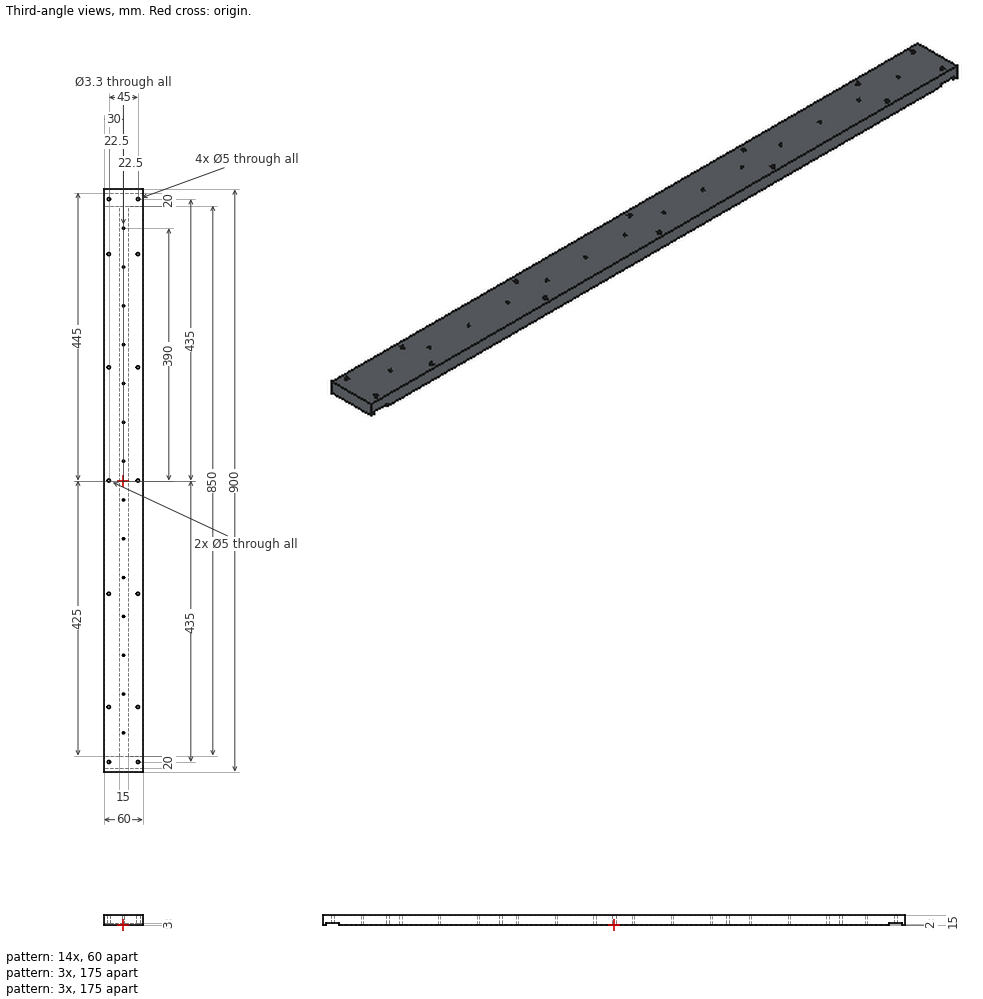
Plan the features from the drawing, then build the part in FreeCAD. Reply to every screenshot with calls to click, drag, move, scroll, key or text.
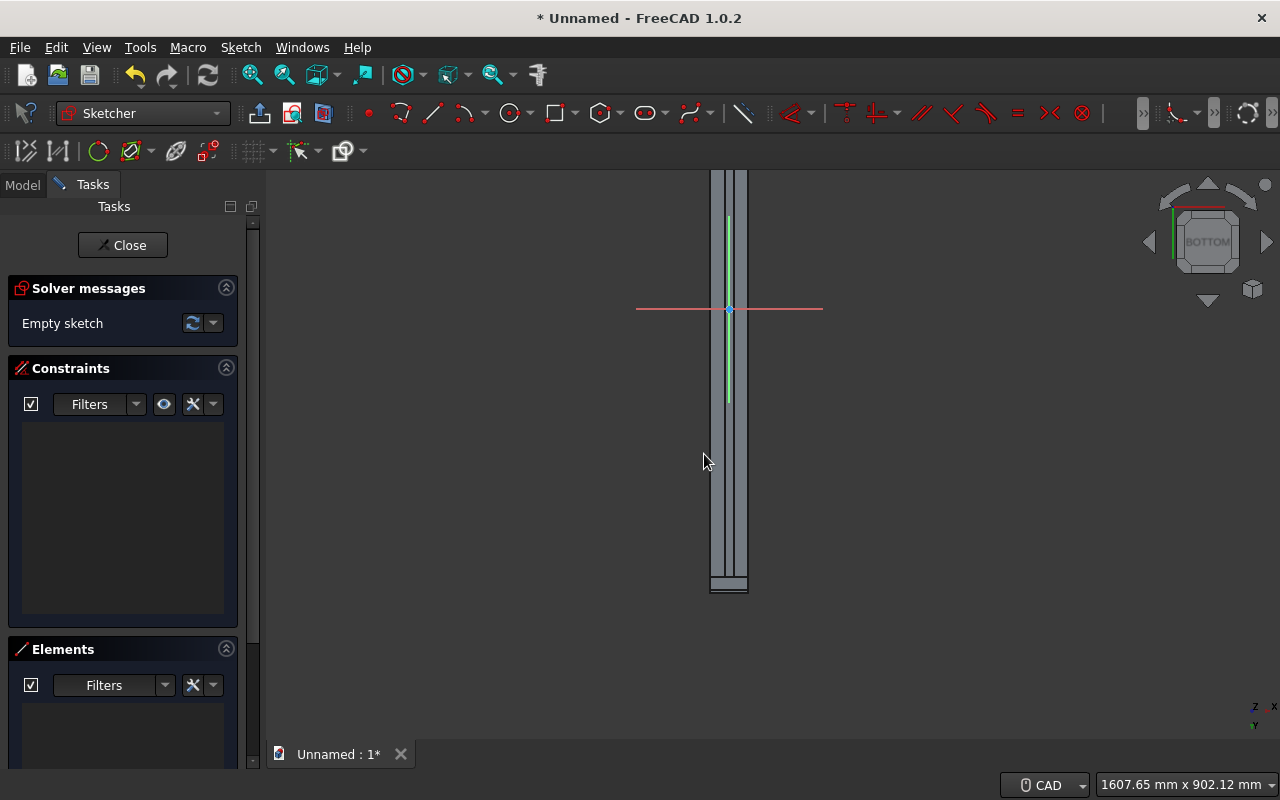
scroll(731, 560, up, 15)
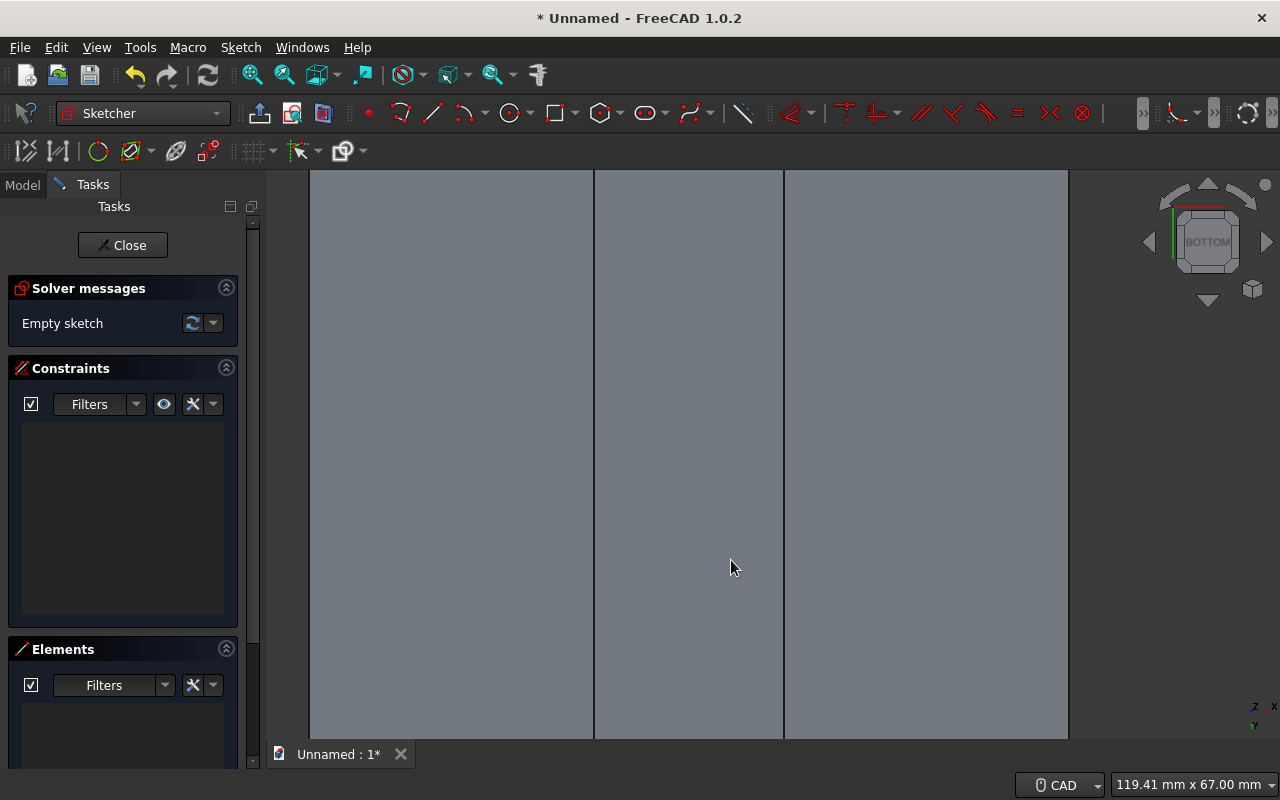
scroll(687, 446, up, 11)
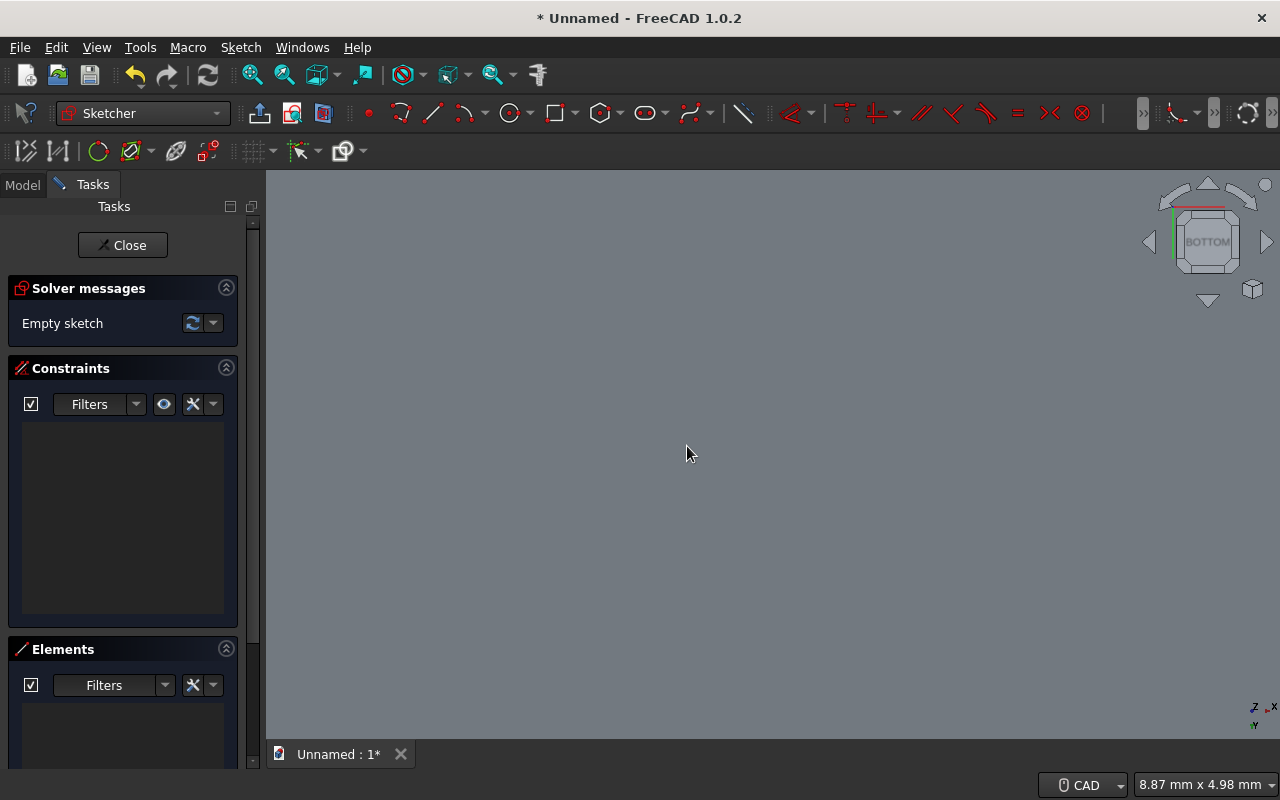
key(g)
key(c)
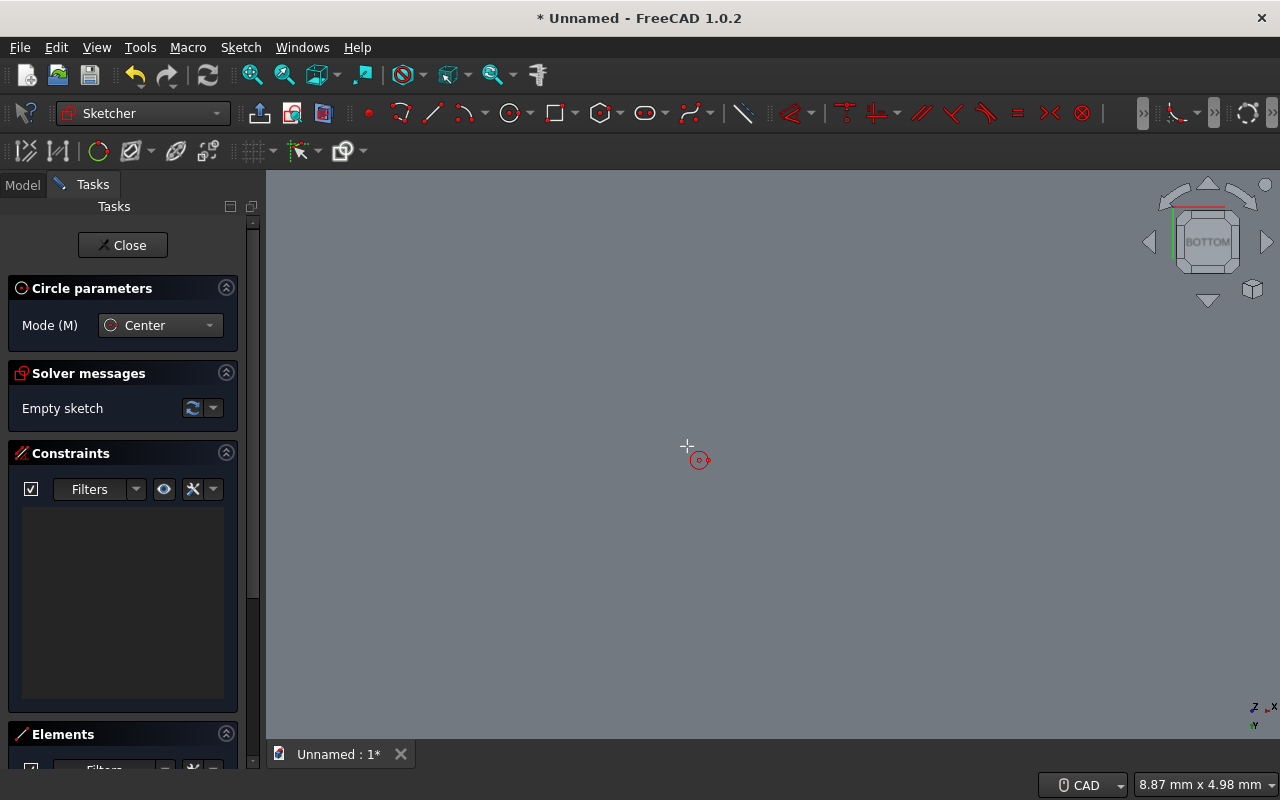
click(705, 449)
move(838, 316)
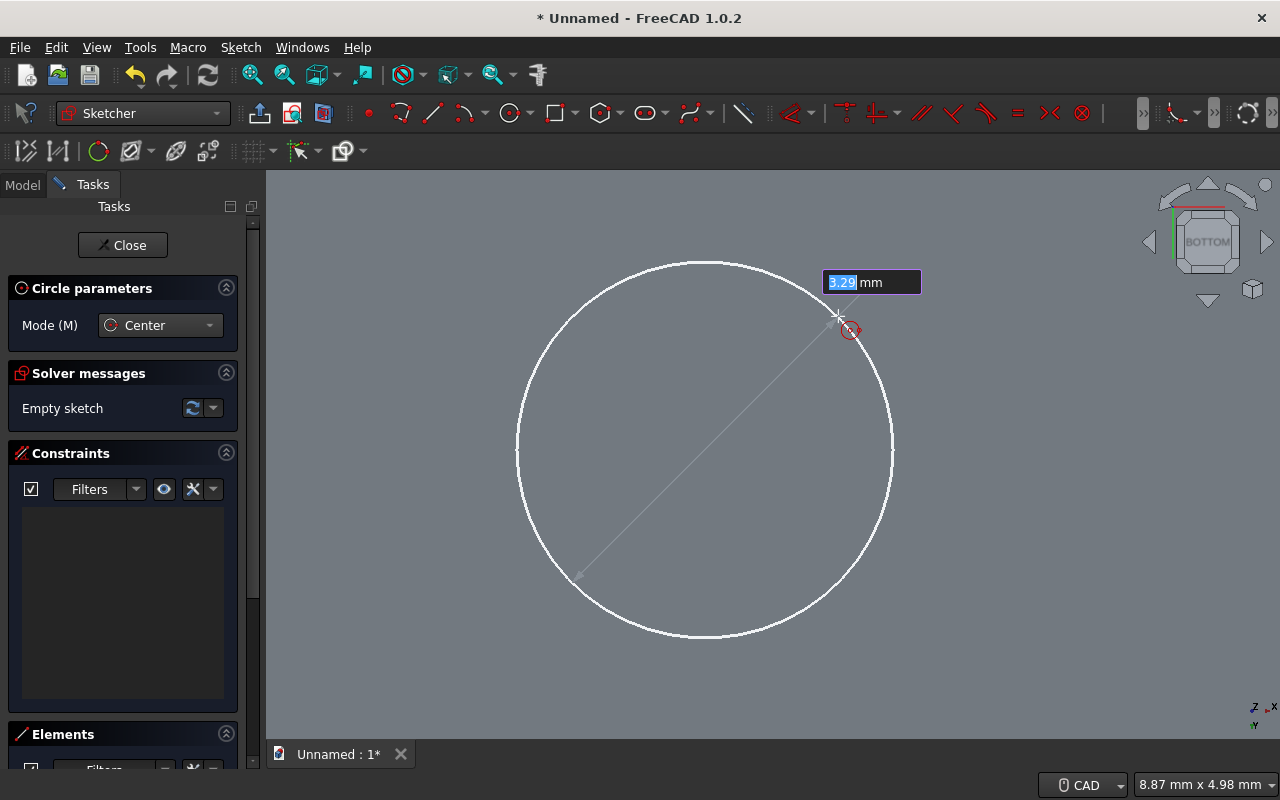
text(3.3)
key(Return)
key(Escape)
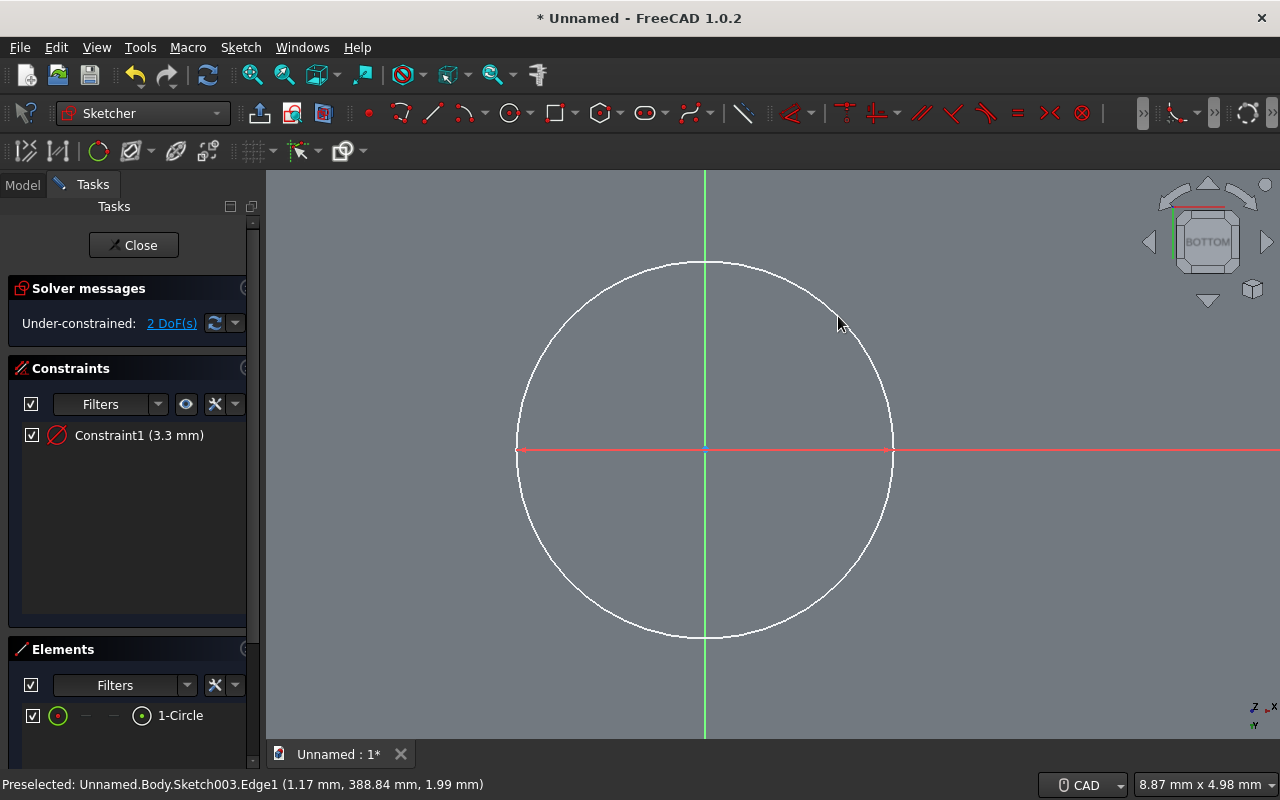
click(705, 450)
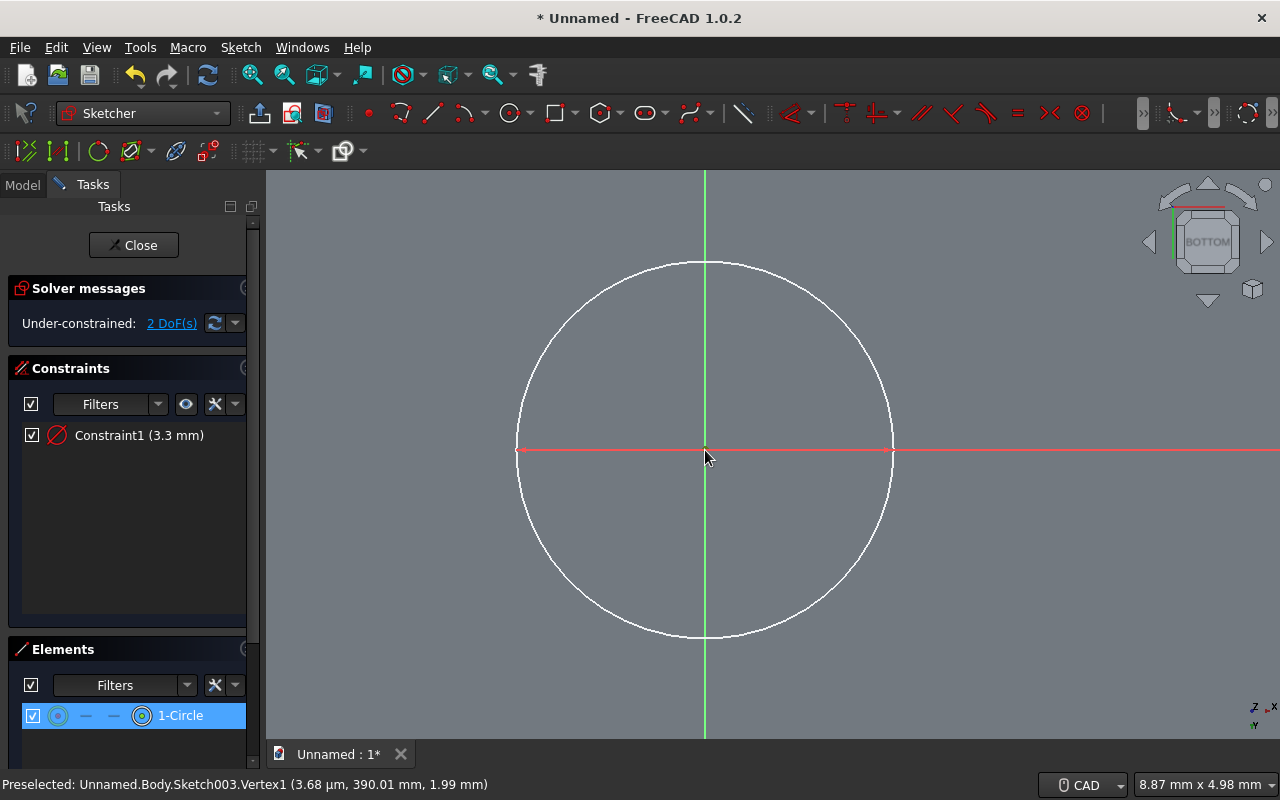
click(705, 674)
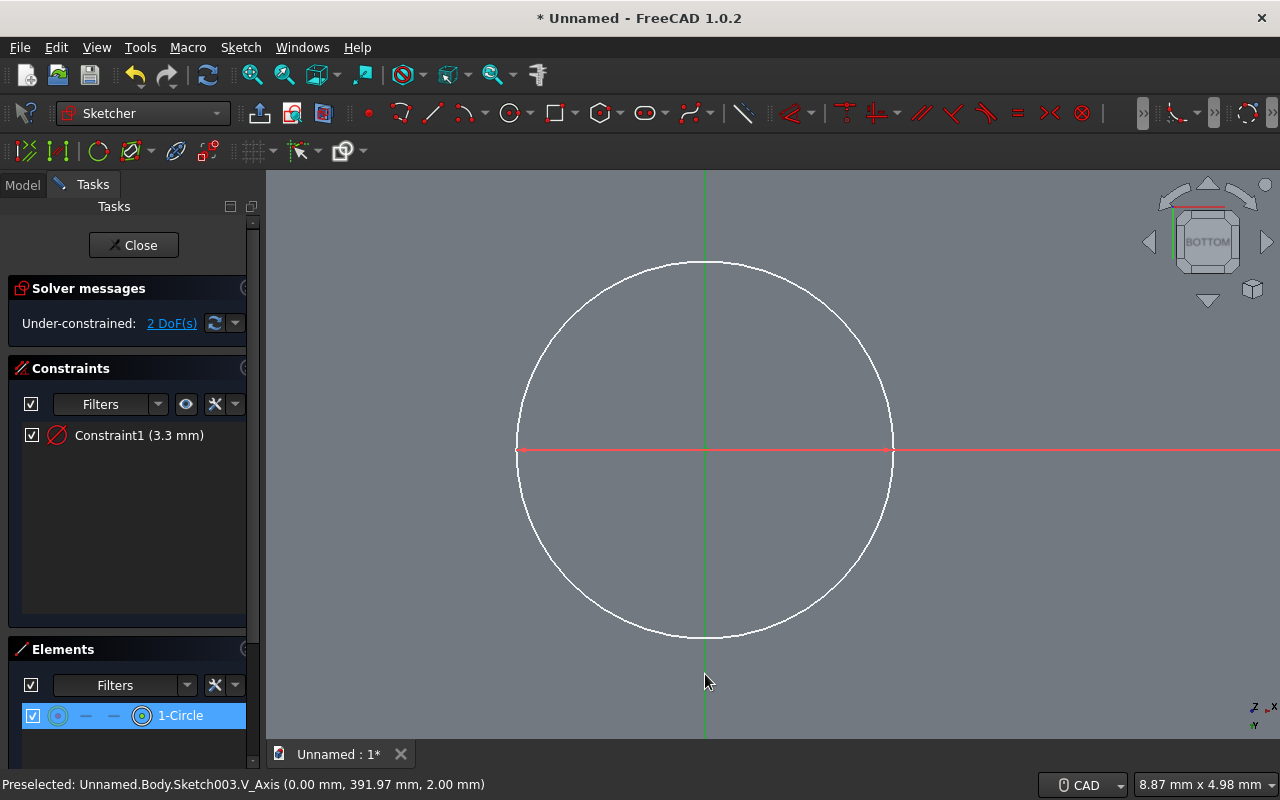
click(846, 114)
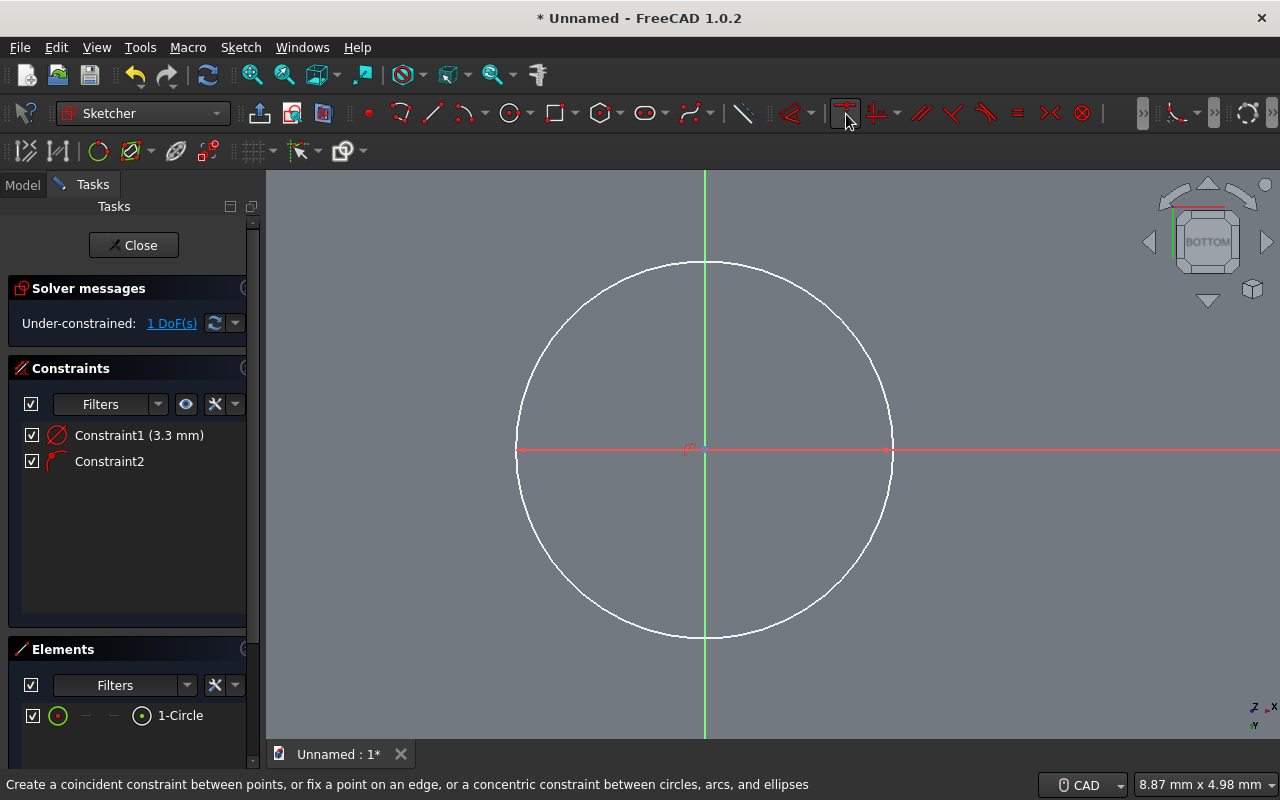
key(d)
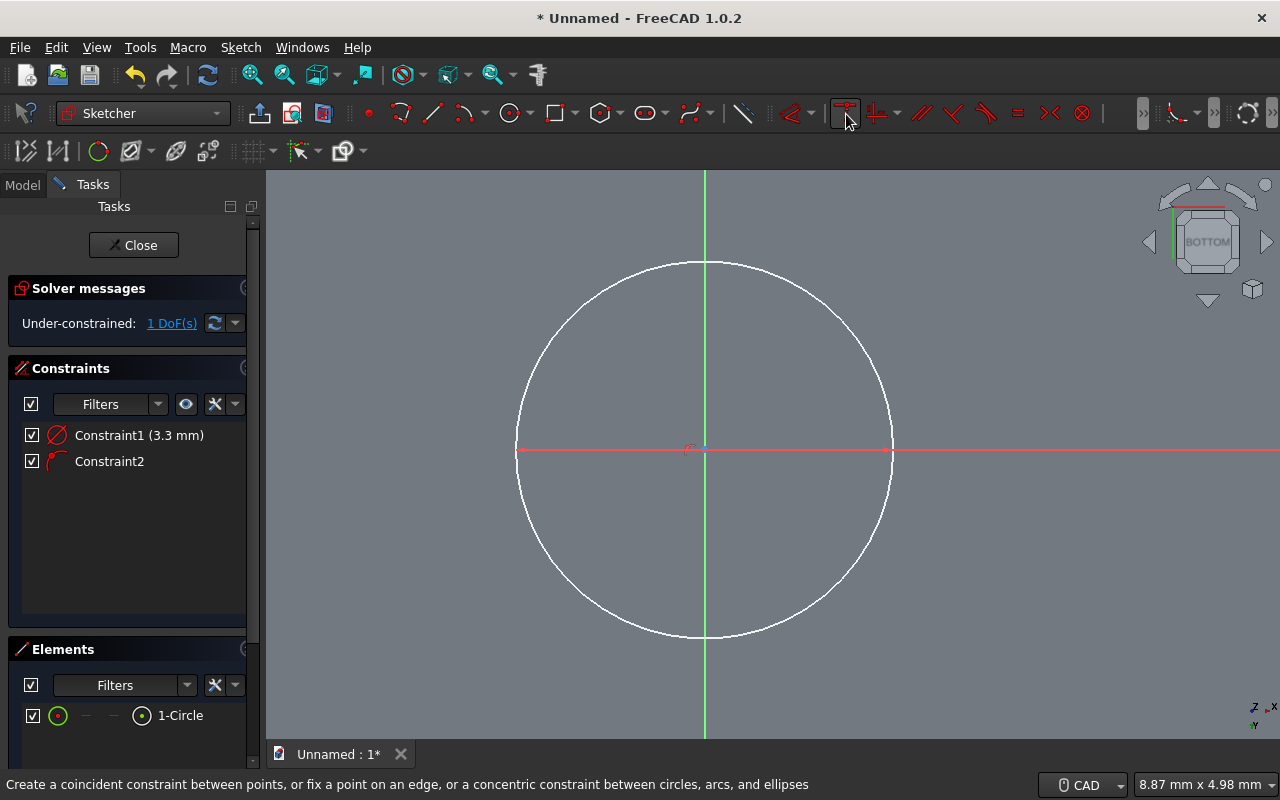
click(705, 450)
click(739, 324)